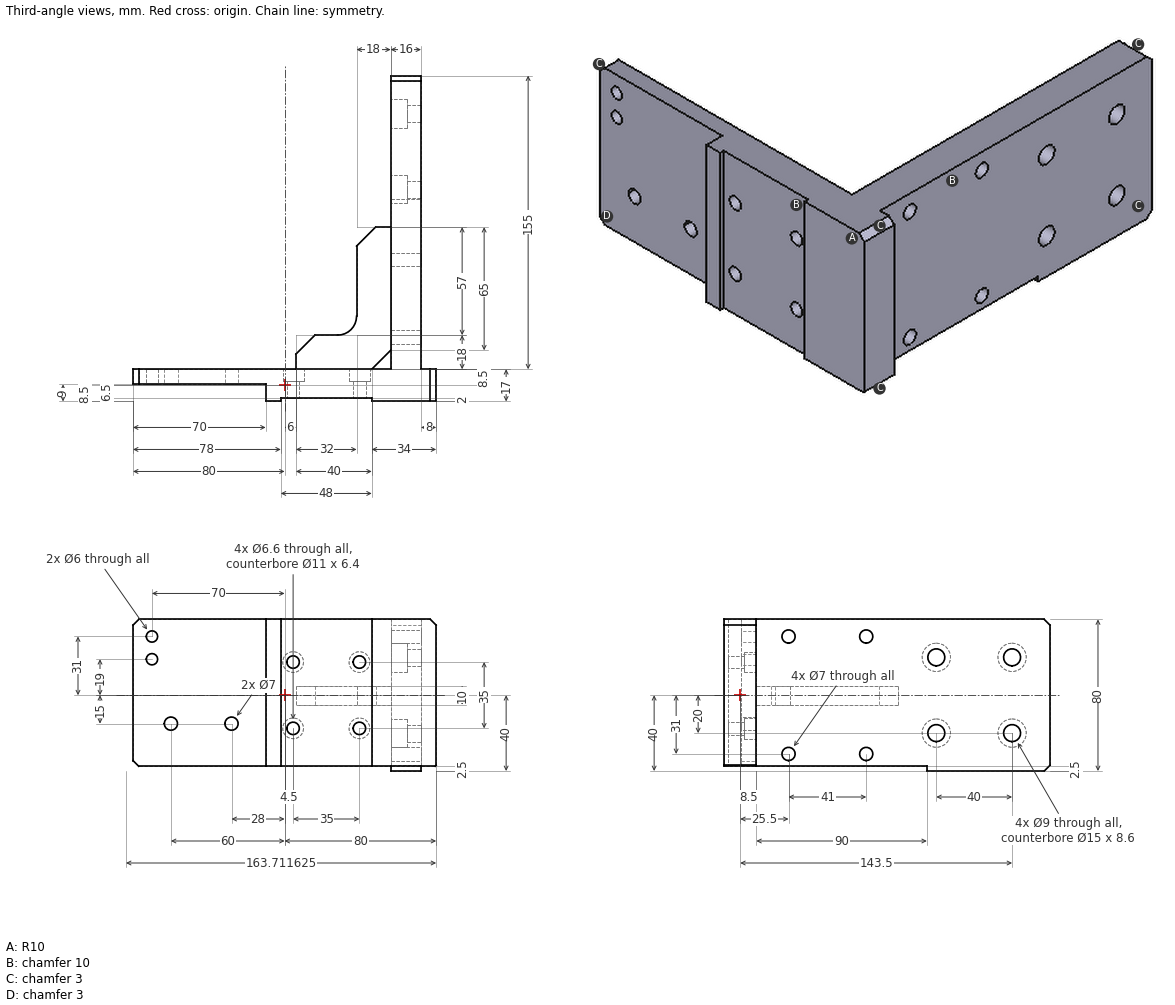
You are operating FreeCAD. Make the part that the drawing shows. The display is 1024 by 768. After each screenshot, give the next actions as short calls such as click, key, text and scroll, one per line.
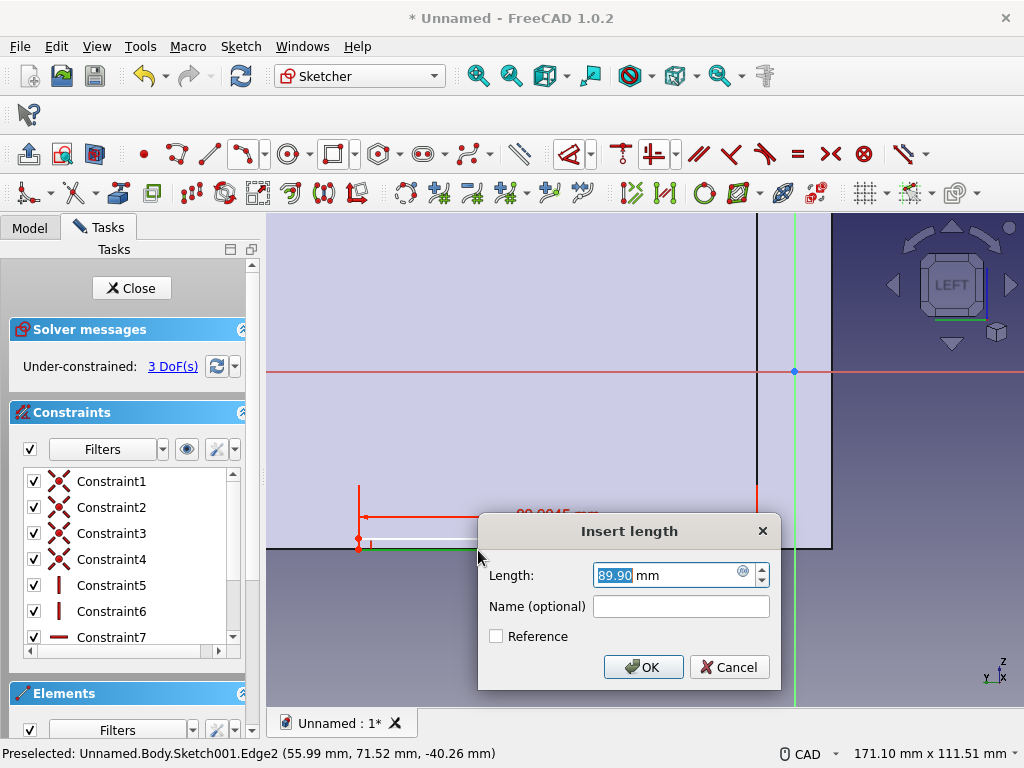
text(90)
key(Return)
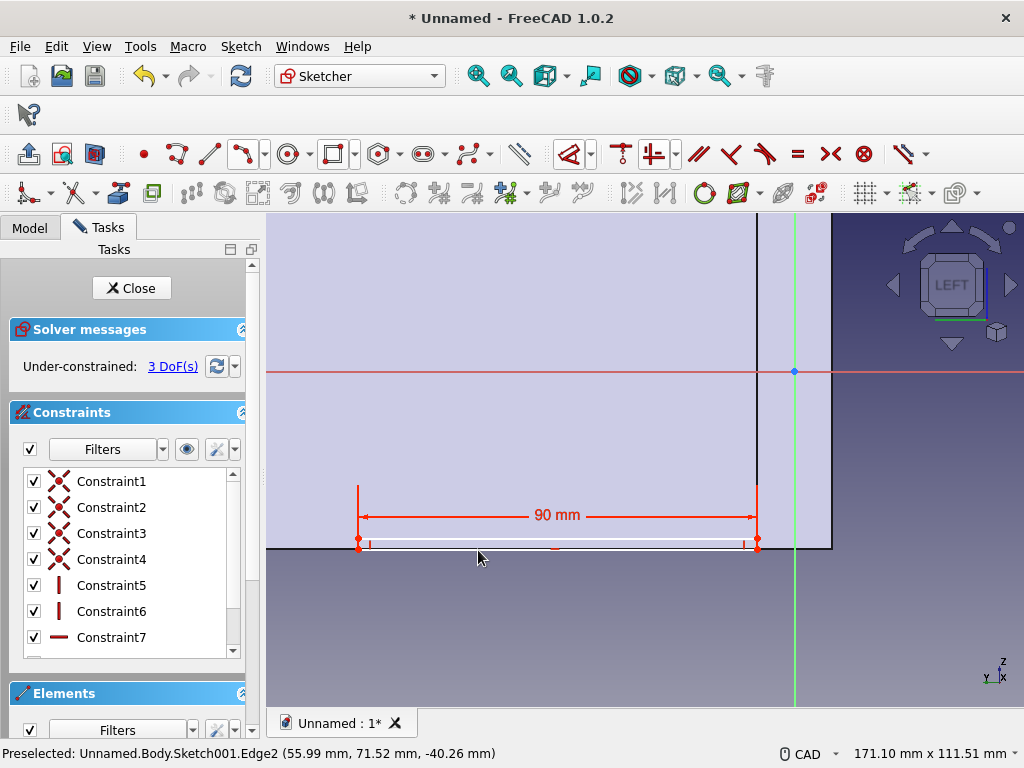
scroll(358, 544, up, 7)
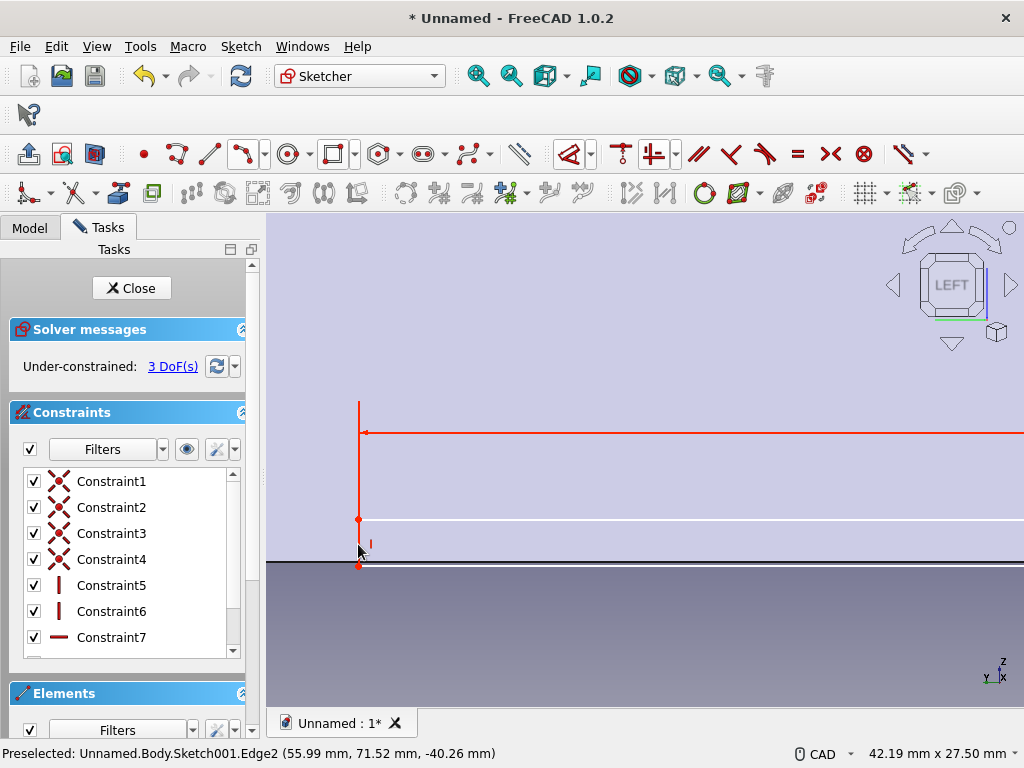
click(359, 543)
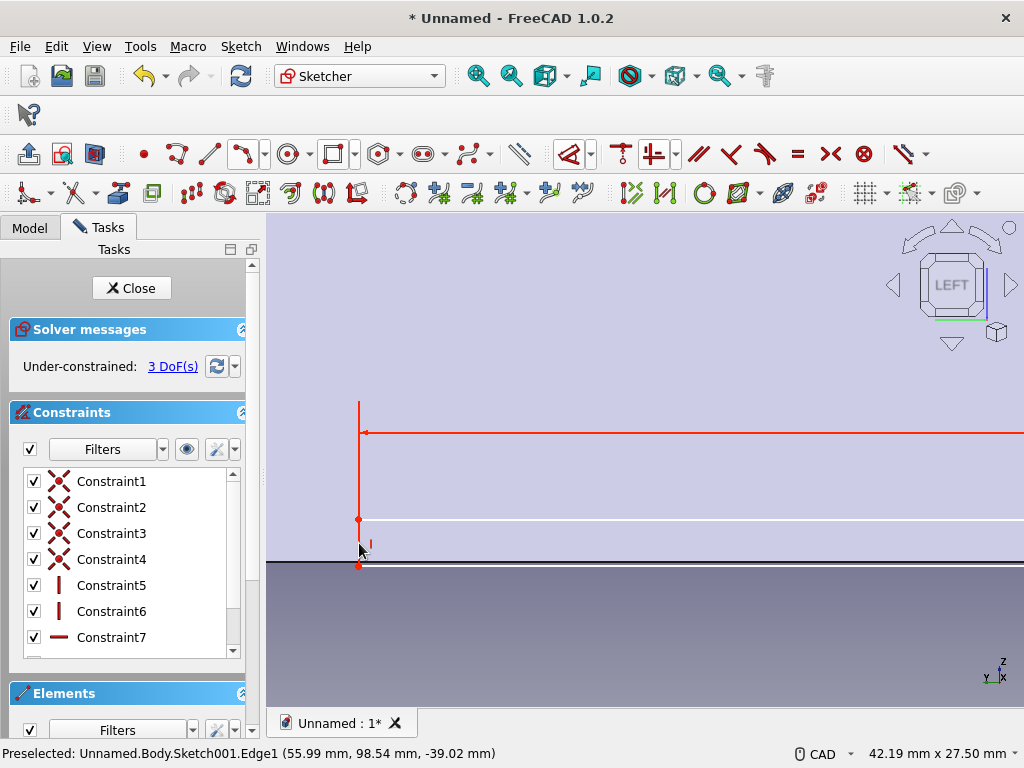
click(590, 154)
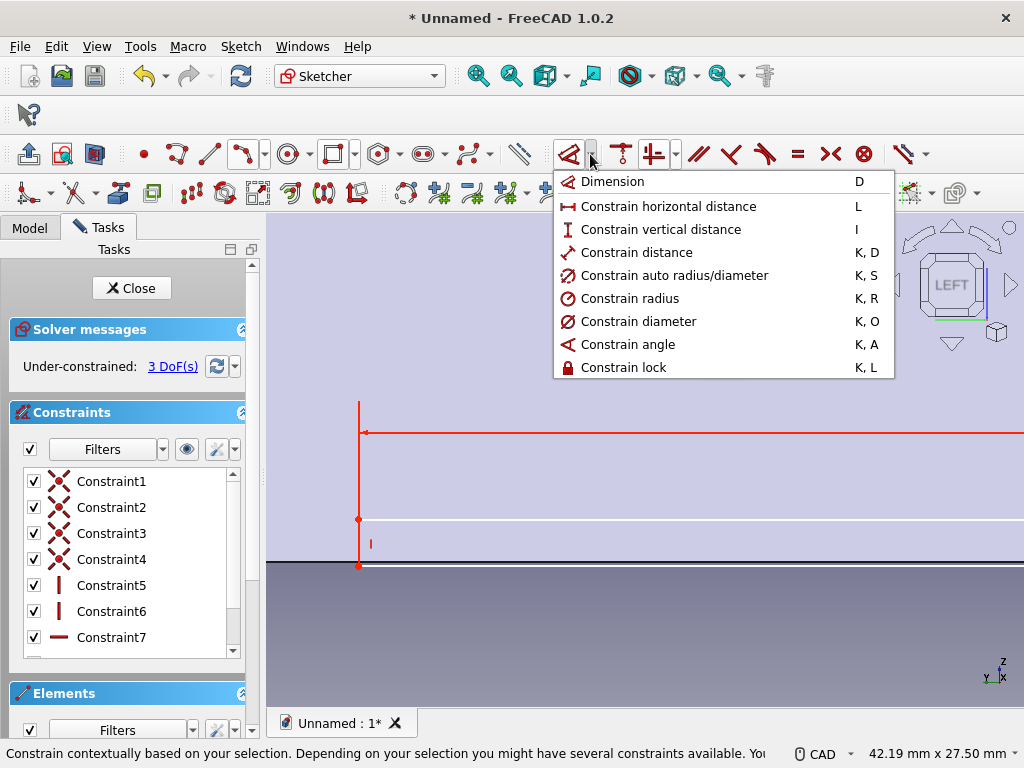
click(724, 230)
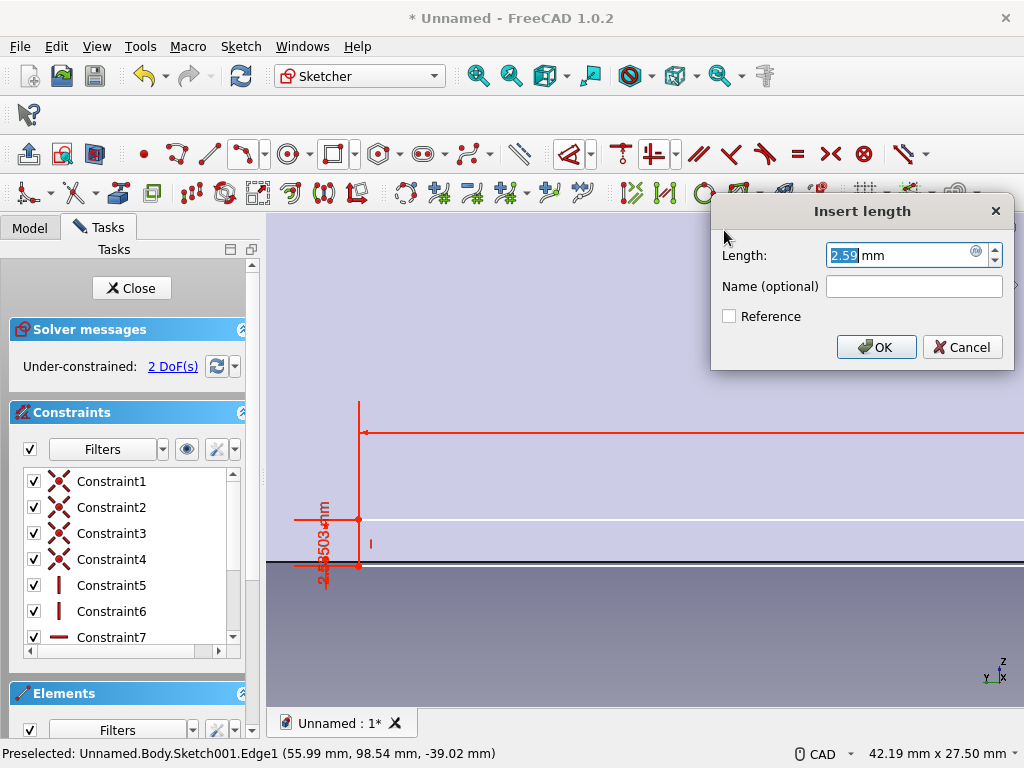
text(2.5)
key(Return)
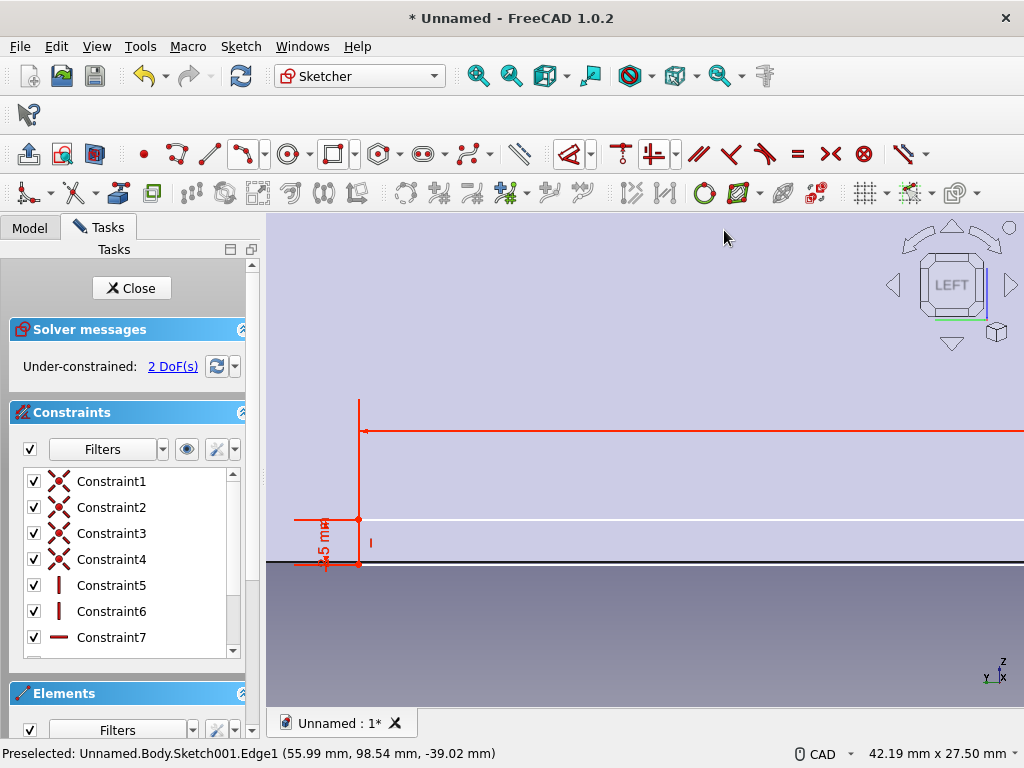
scroll(358, 544, down, 7)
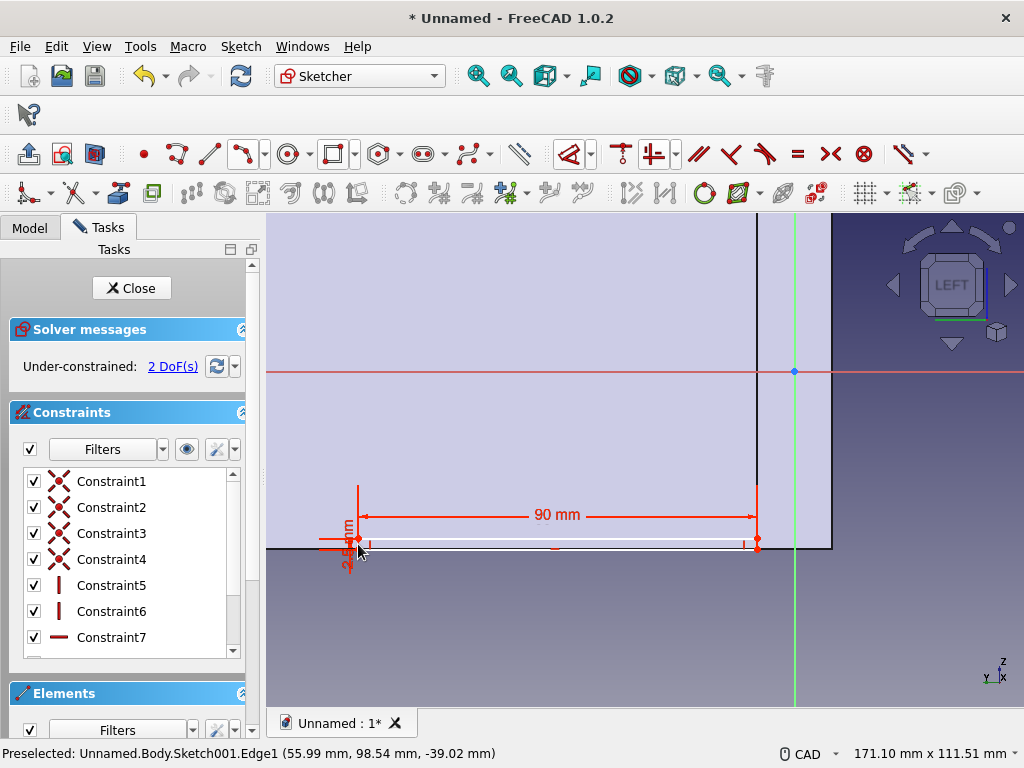
click(358, 550)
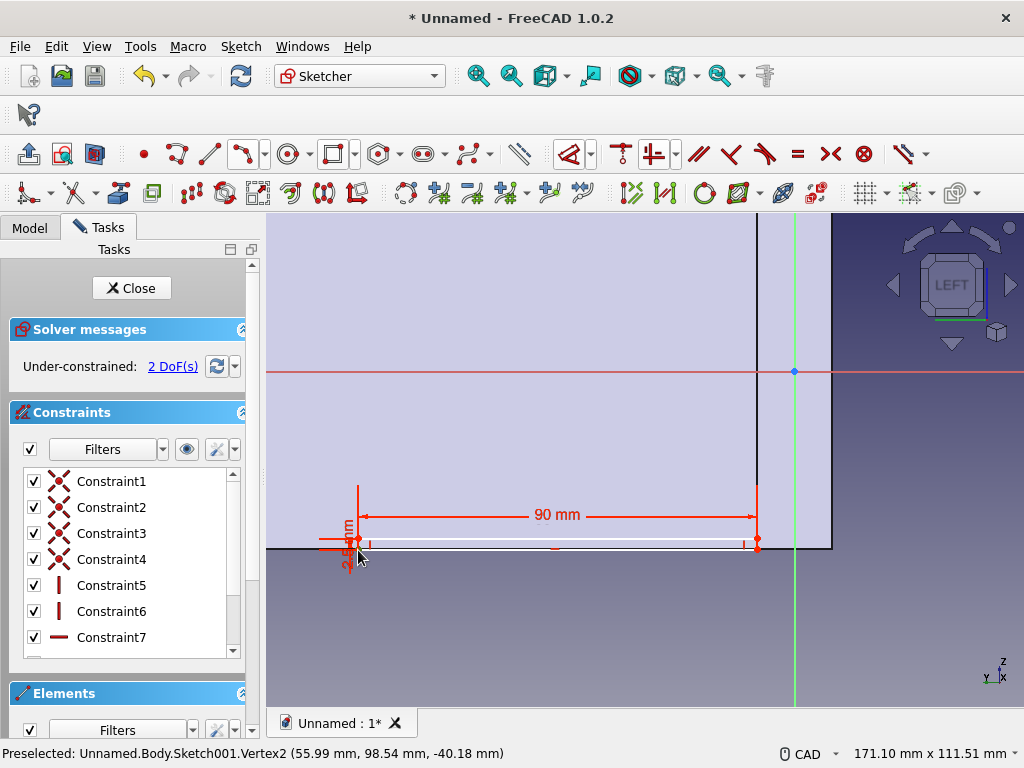
click(590, 154)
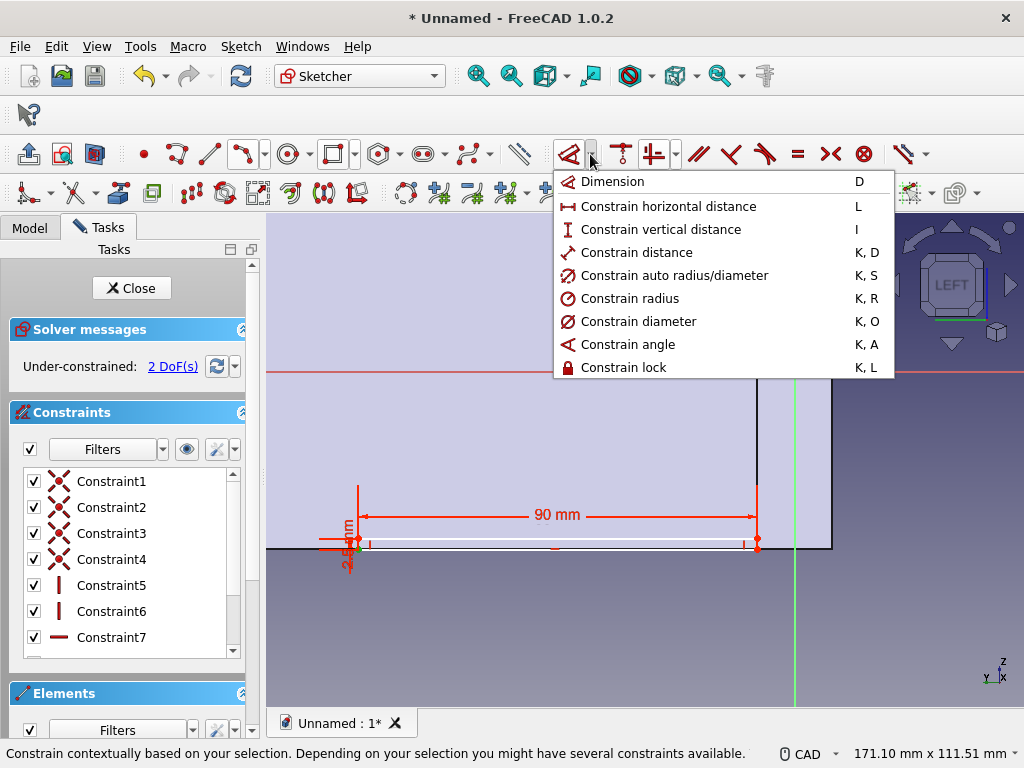
click(724, 230)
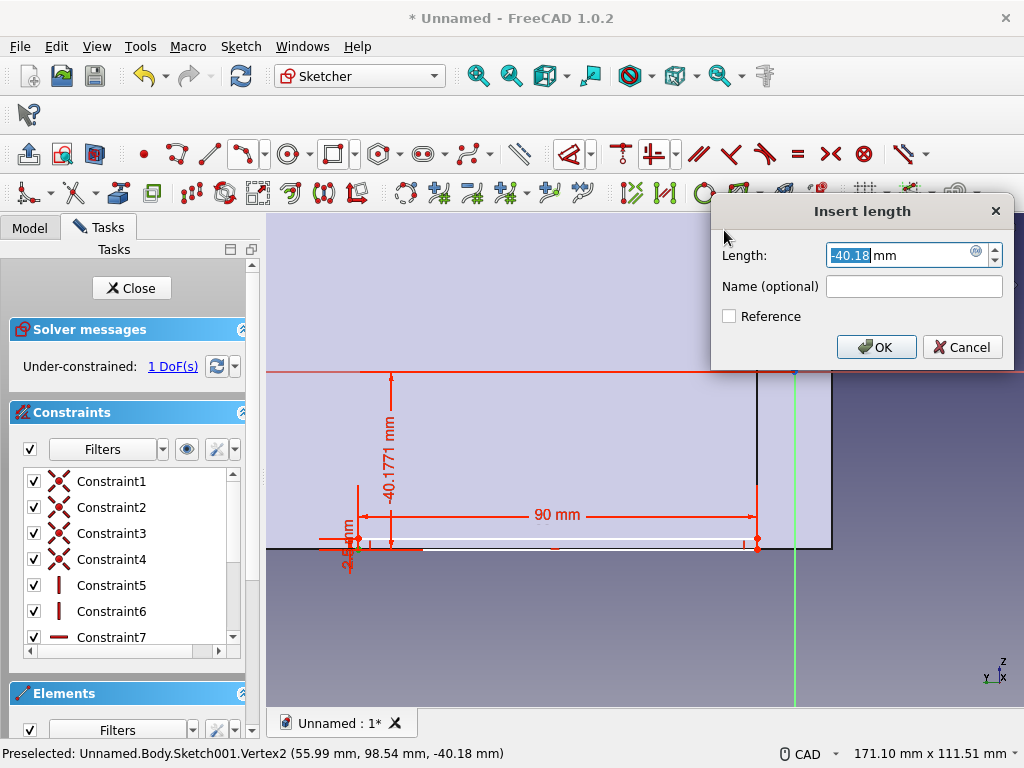
text(-40)
key(Return)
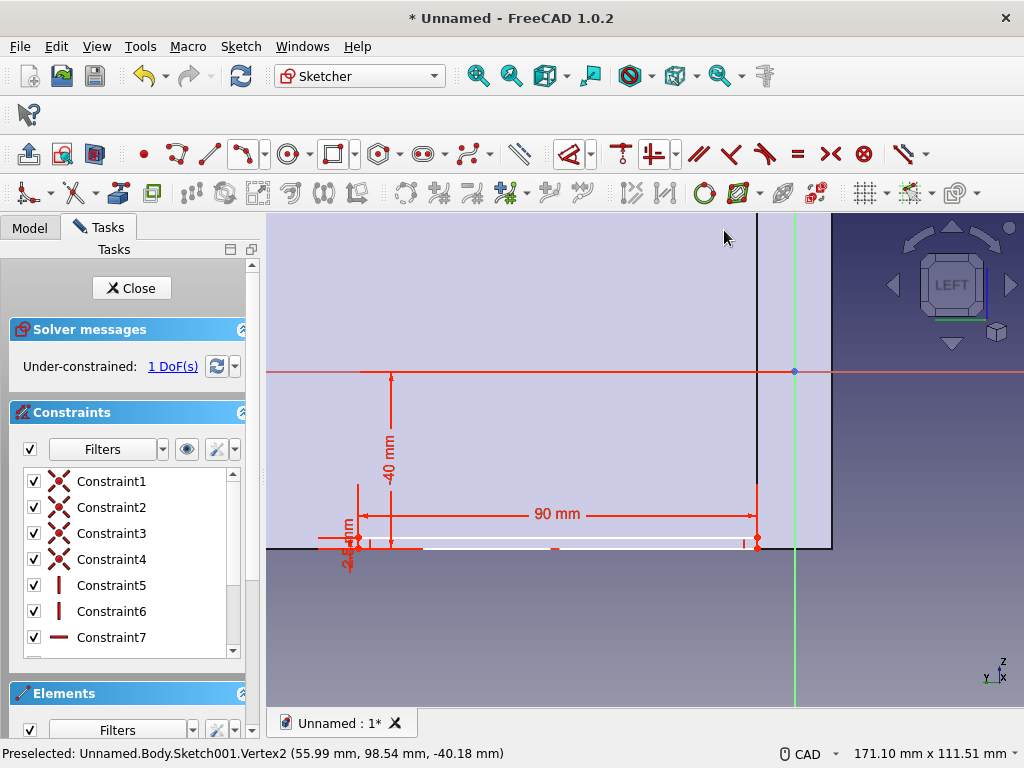
click(757, 549)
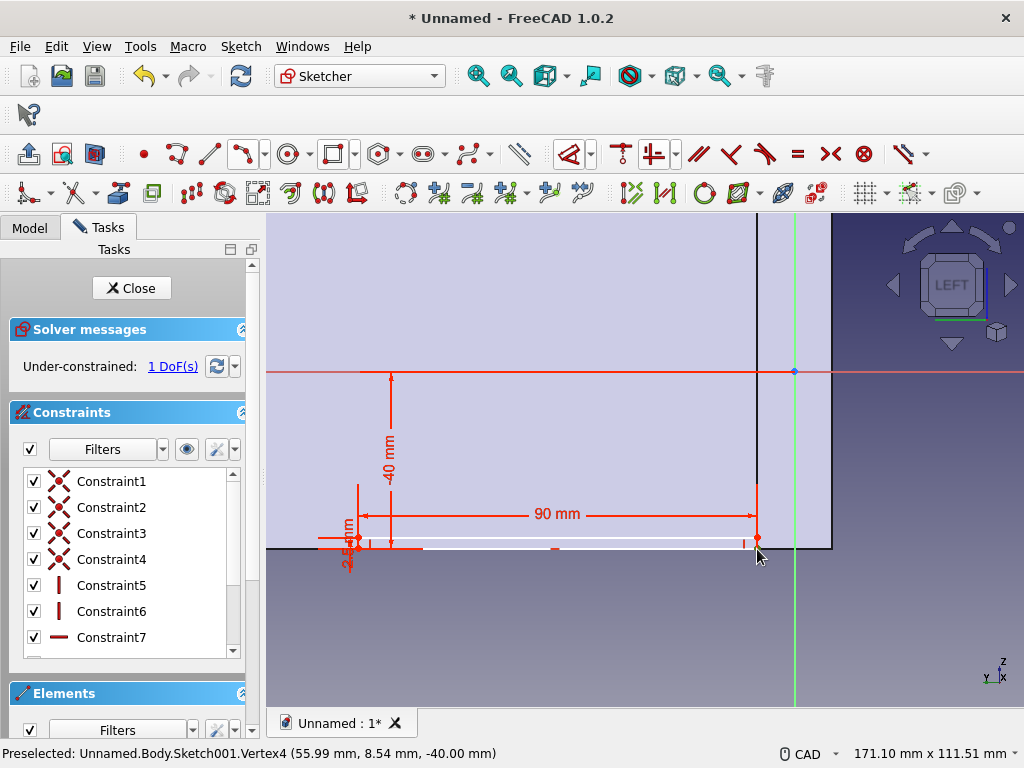
click(590, 154)